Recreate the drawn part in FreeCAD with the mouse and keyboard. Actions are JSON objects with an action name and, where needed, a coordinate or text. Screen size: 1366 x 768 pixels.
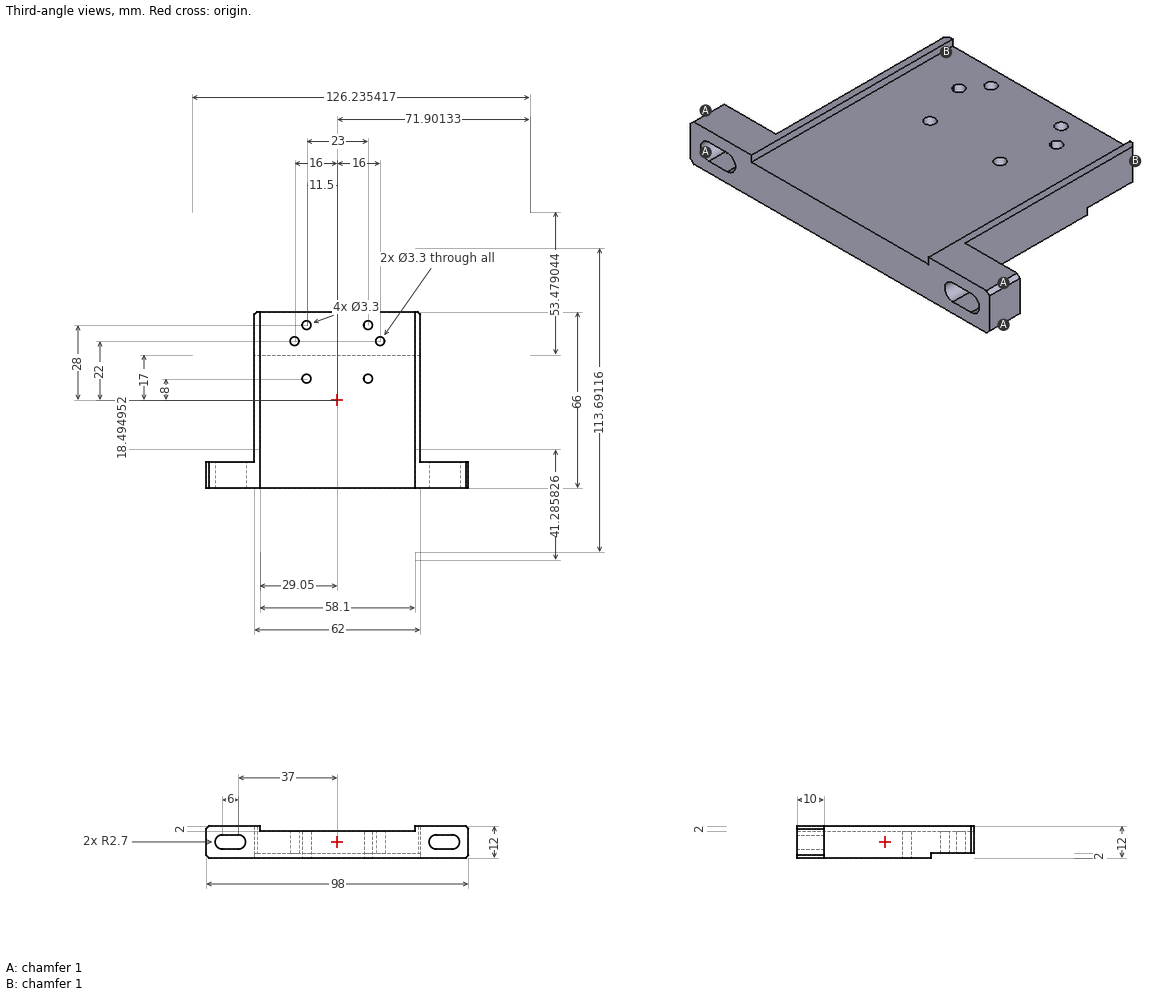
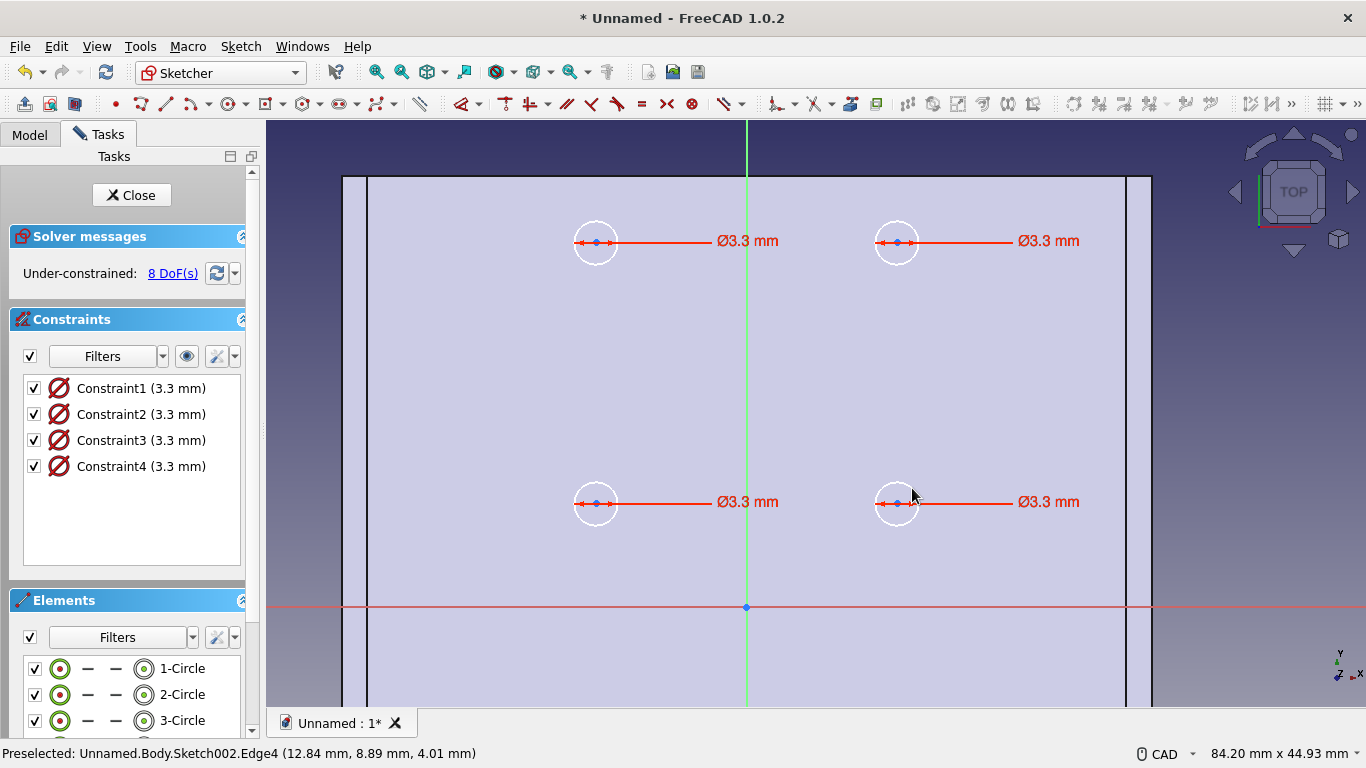
{"action": "left_click", "coordinate": [596, 243]}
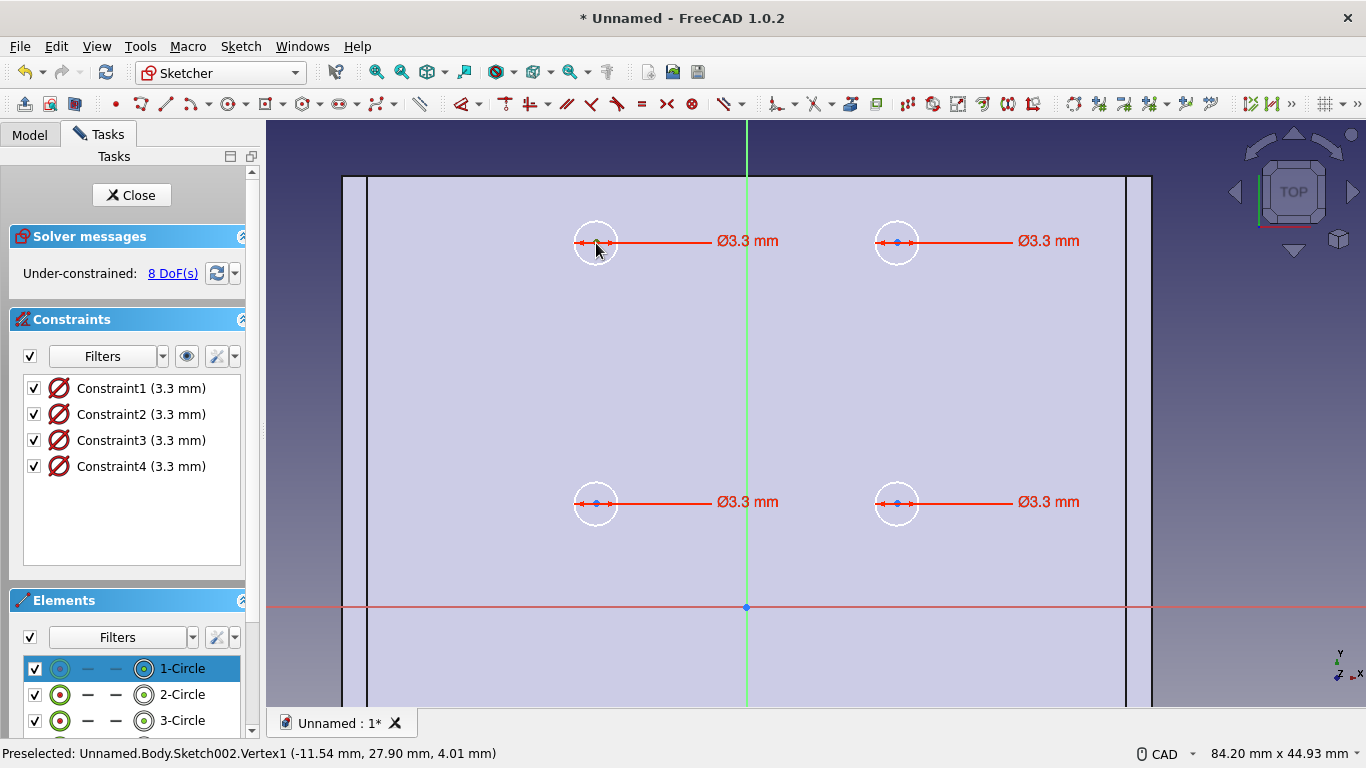
{"action": "left_click", "coordinate": [897, 243]}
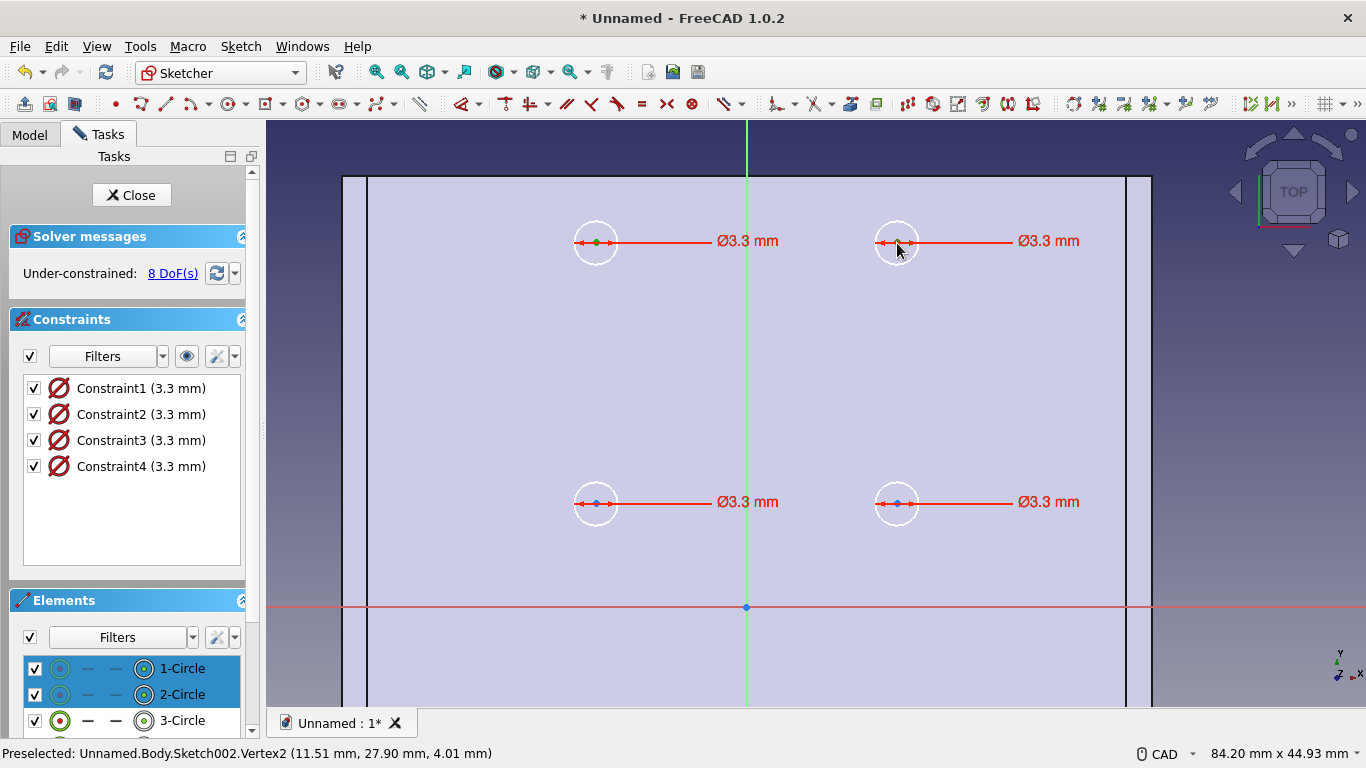
{"action": "key", "text": "h"}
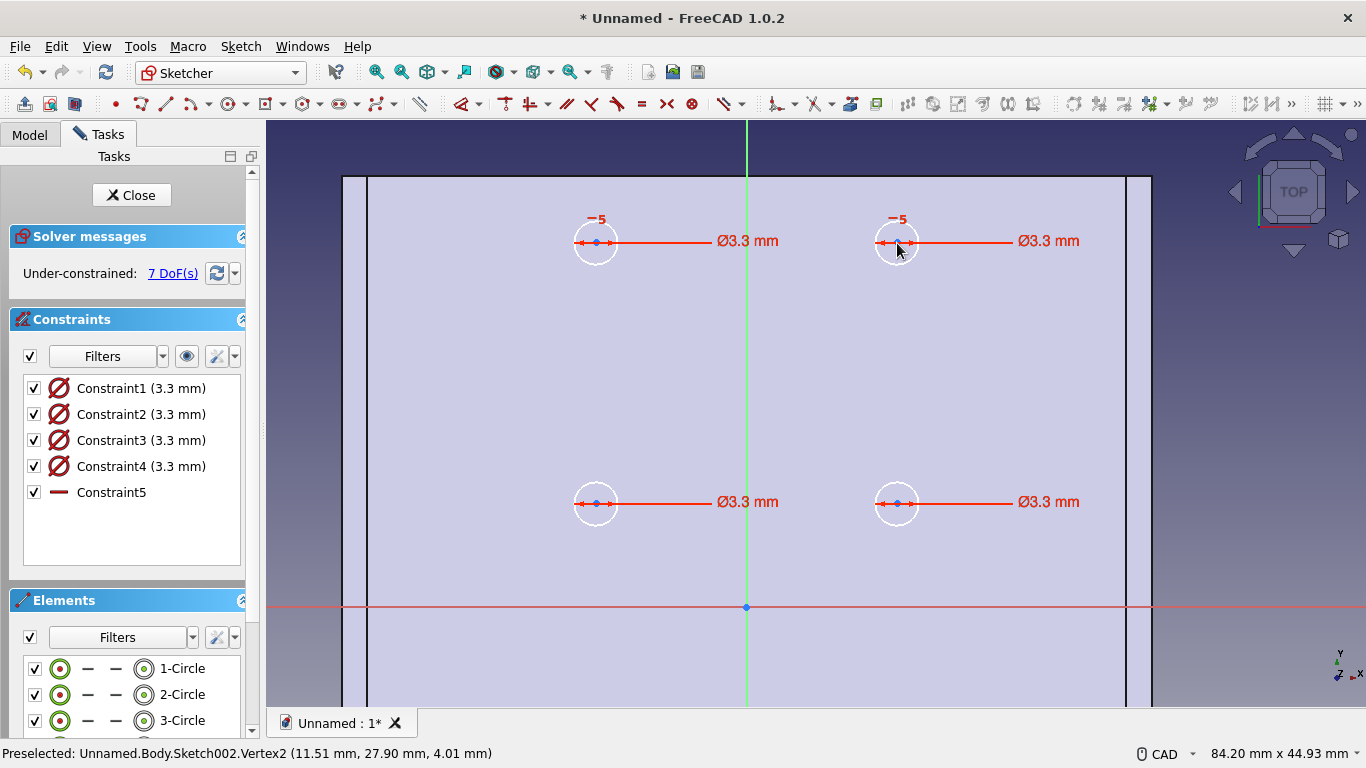
{"action": "left_click", "coordinate": [596, 243]}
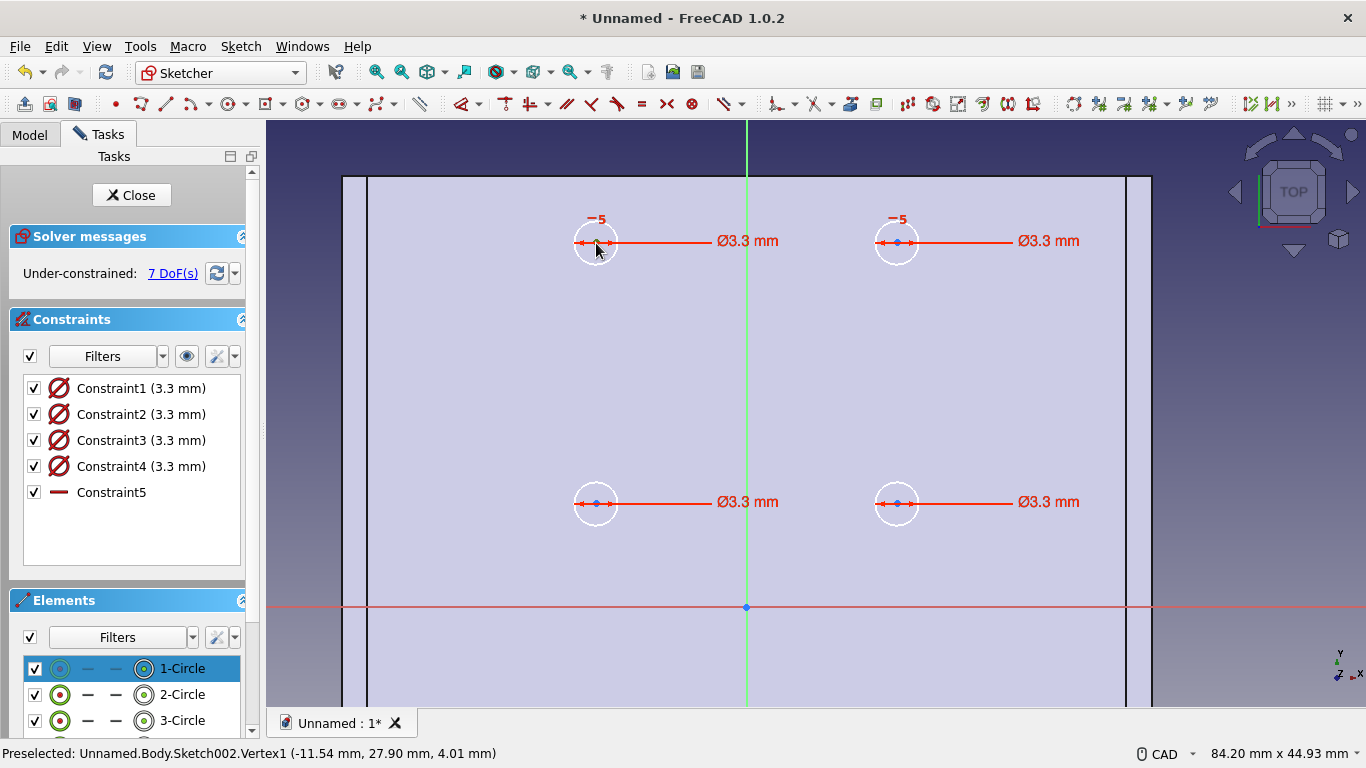
{"action": "left_click", "coordinate": [596, 504]}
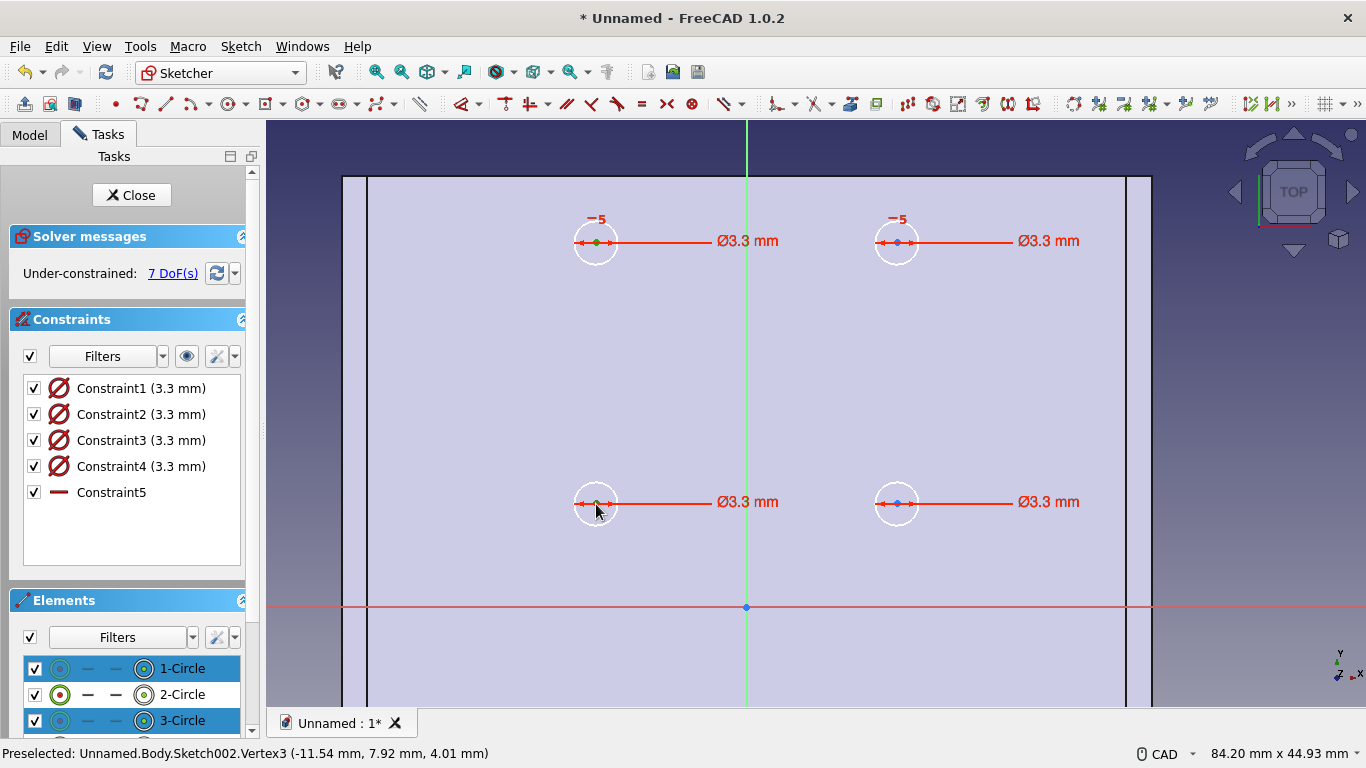
{"action": "key", "text": "v"}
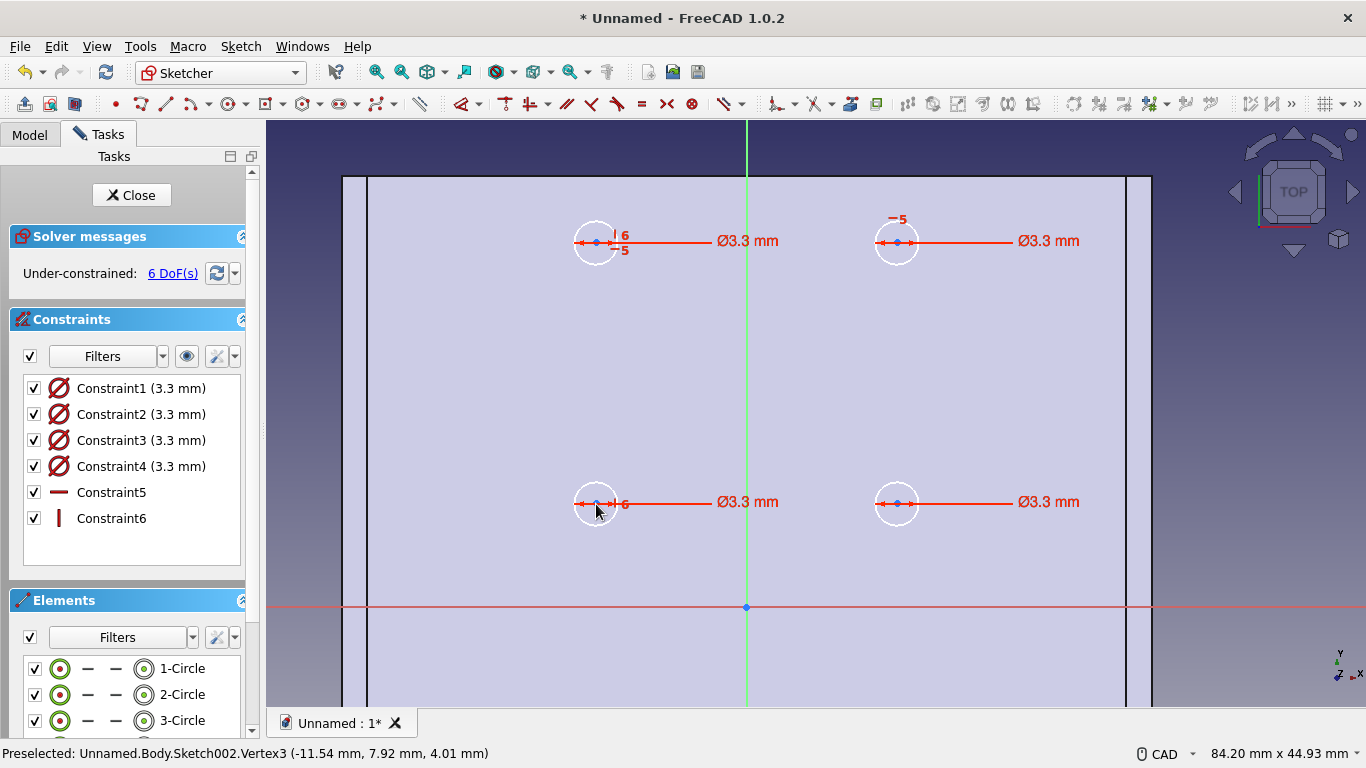
{"action": "left_click", "coordinate": [897, 243]}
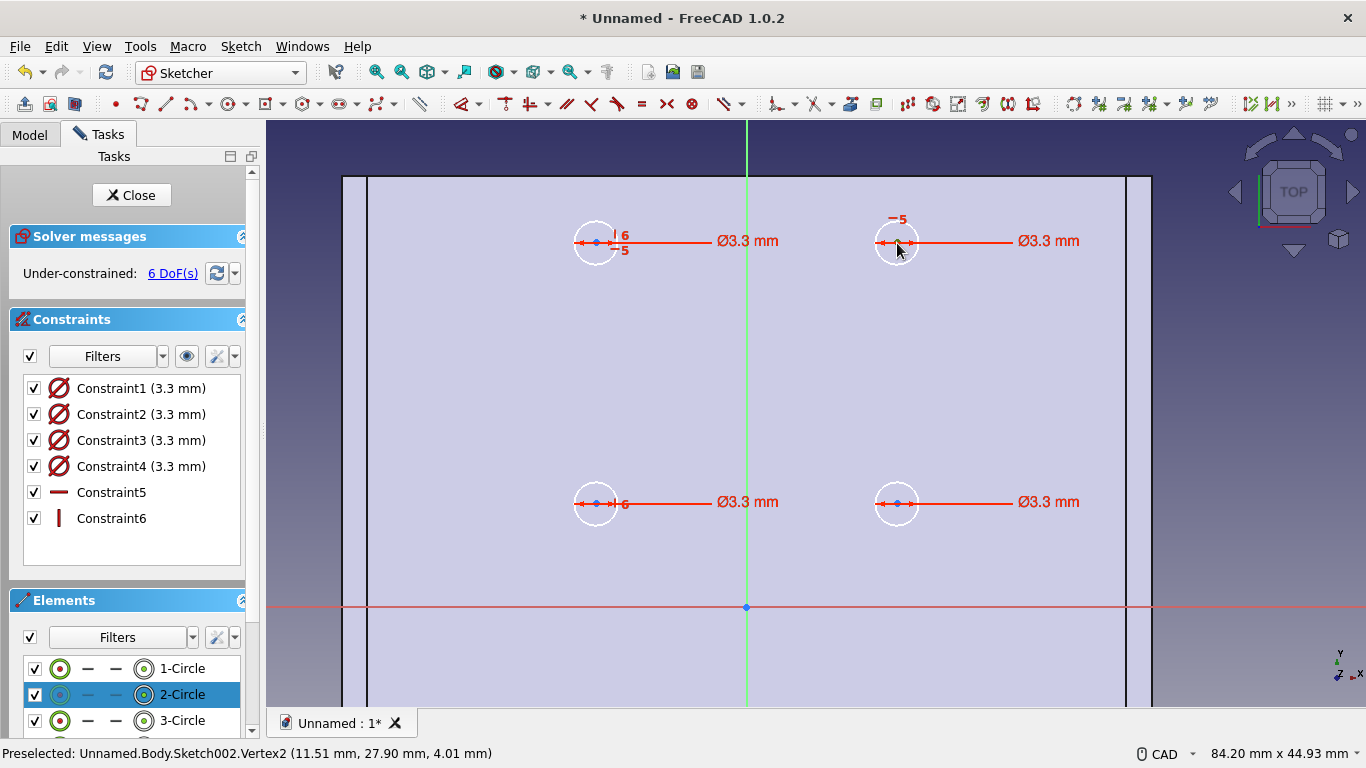
{"action": "left_click", "coordinate": [897, 504]}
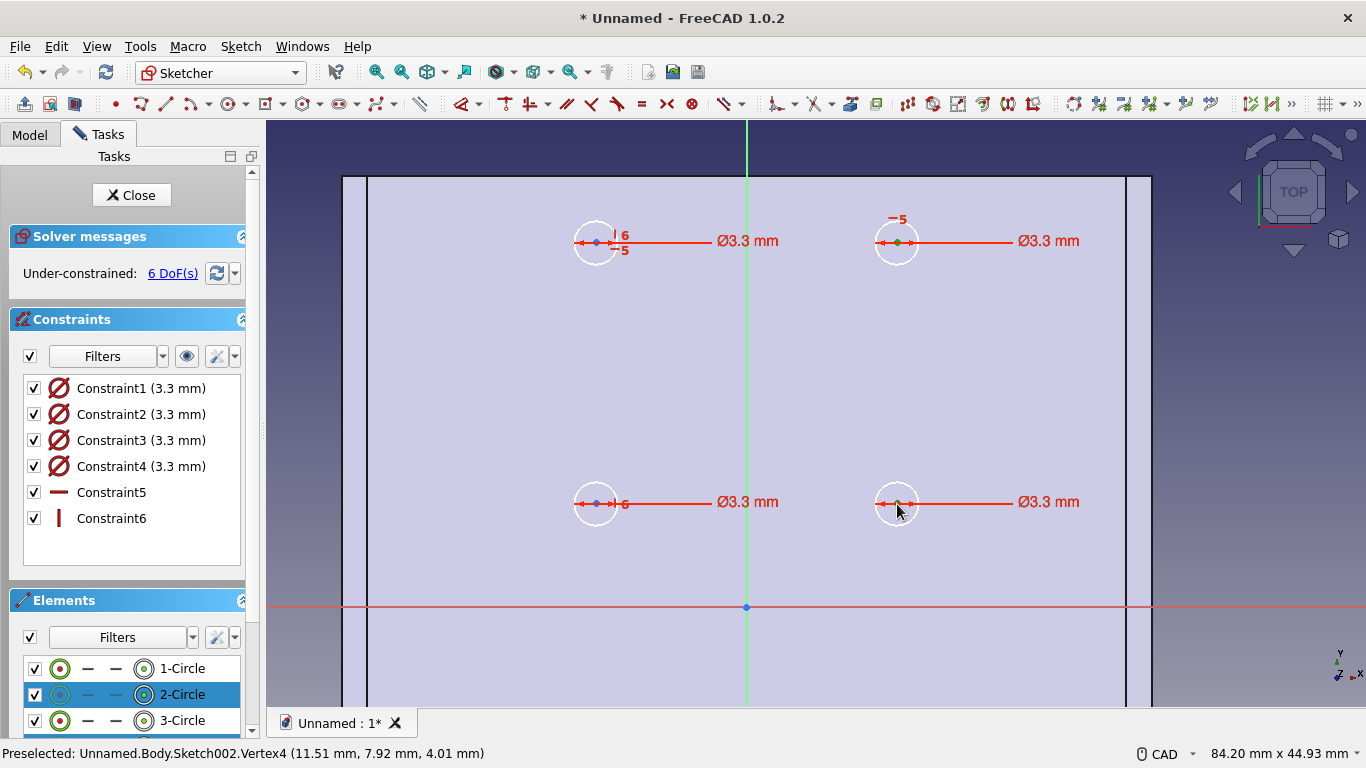
{"action": "key", "text": "v"}